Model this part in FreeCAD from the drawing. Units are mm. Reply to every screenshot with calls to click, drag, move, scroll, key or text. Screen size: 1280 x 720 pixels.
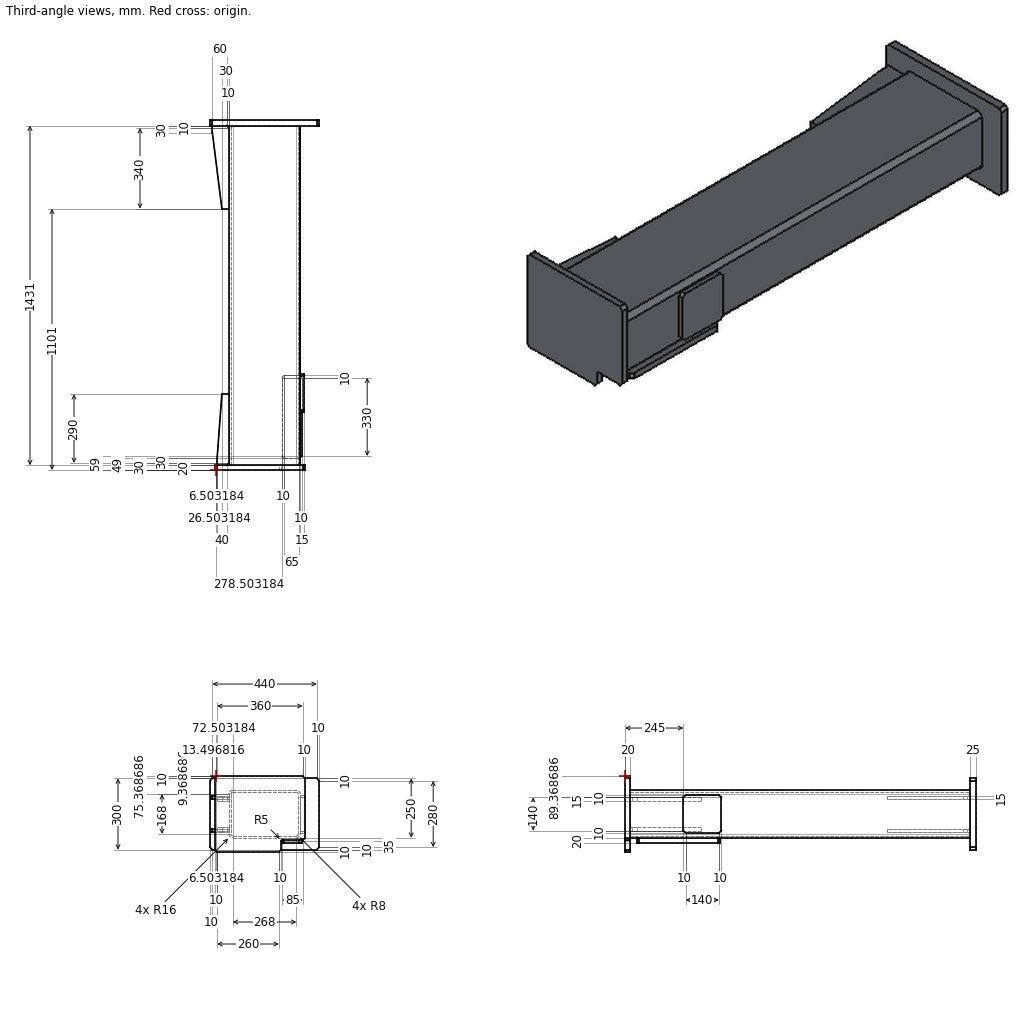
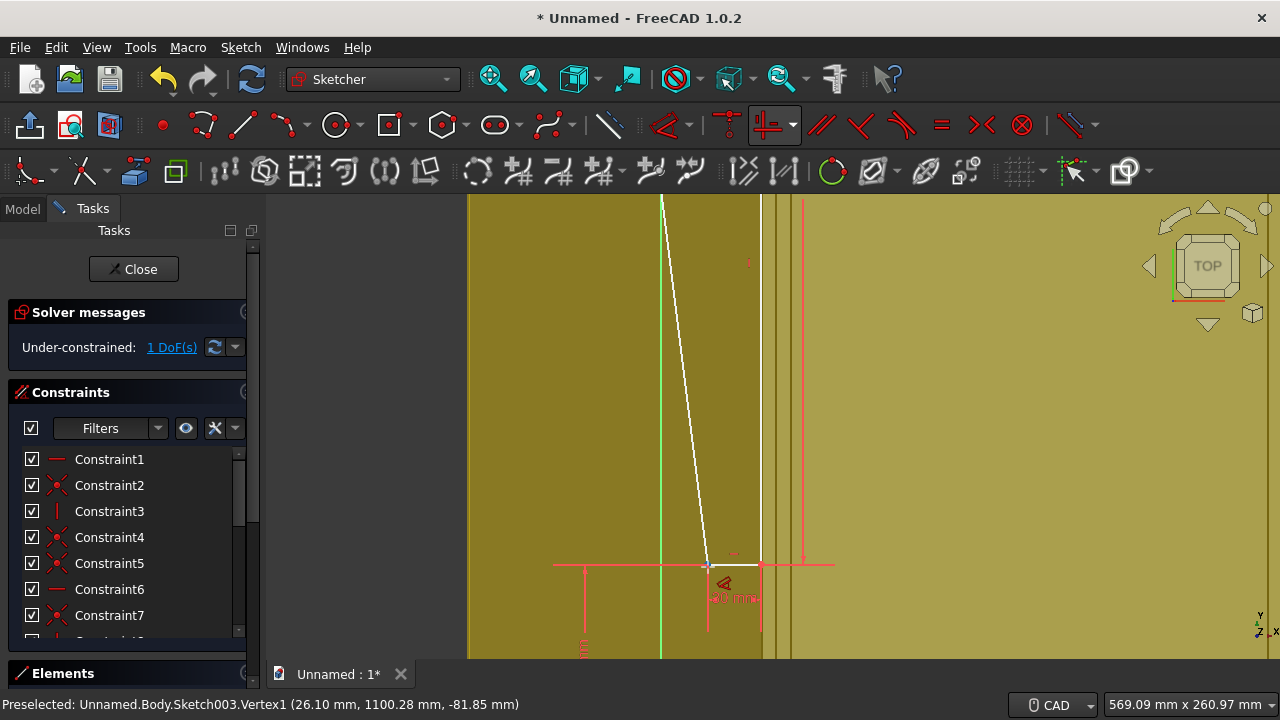
click(708, 565)
click(685, 531)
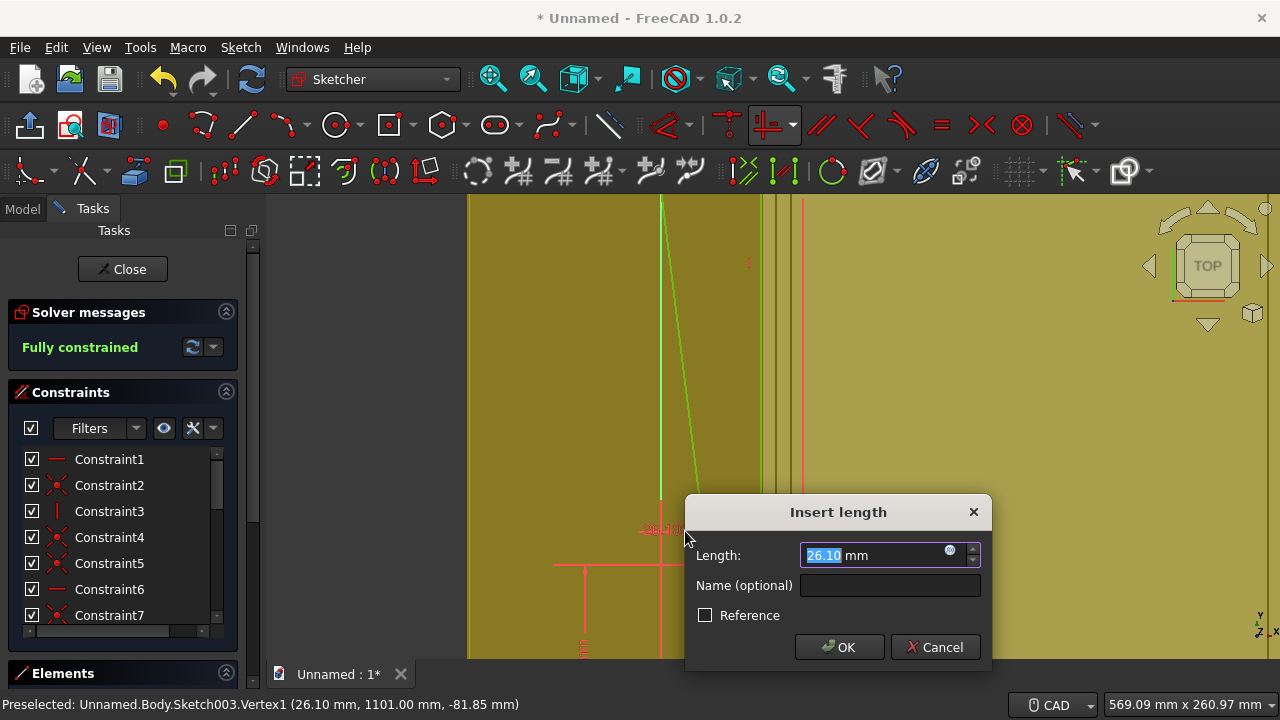
text(26.503184)
key(Return)
key(Escape)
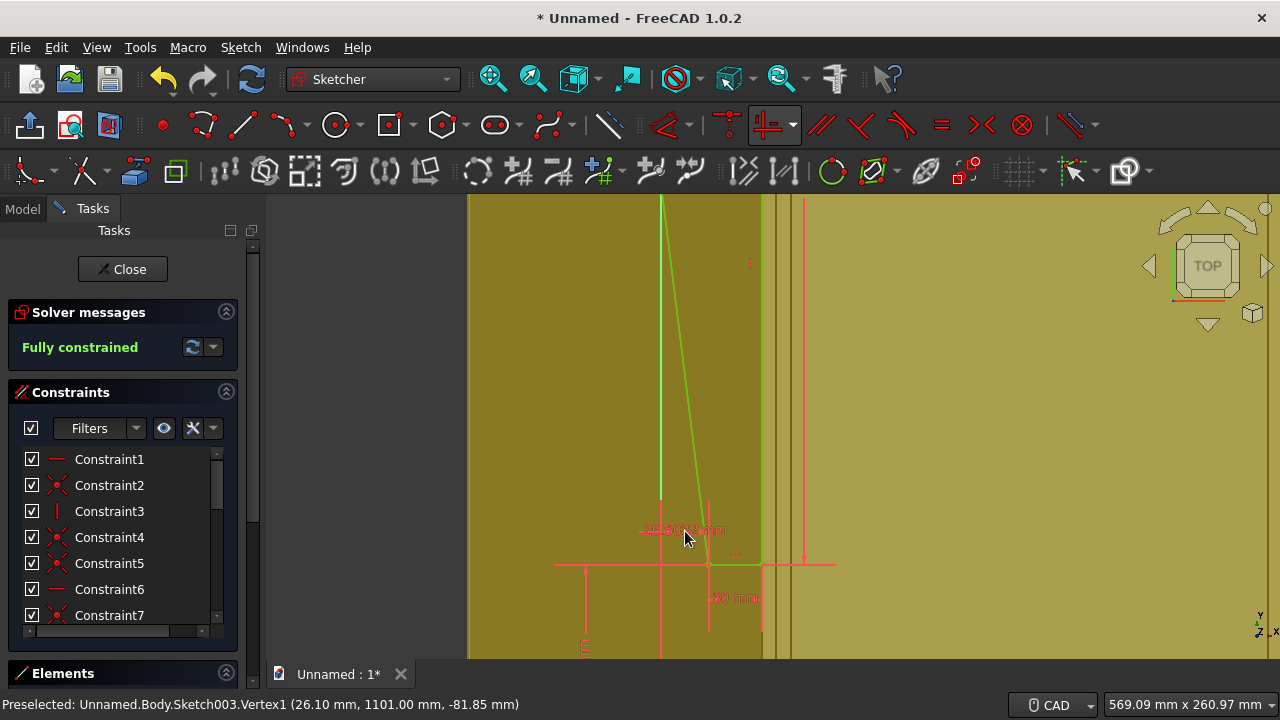
click(123, 269)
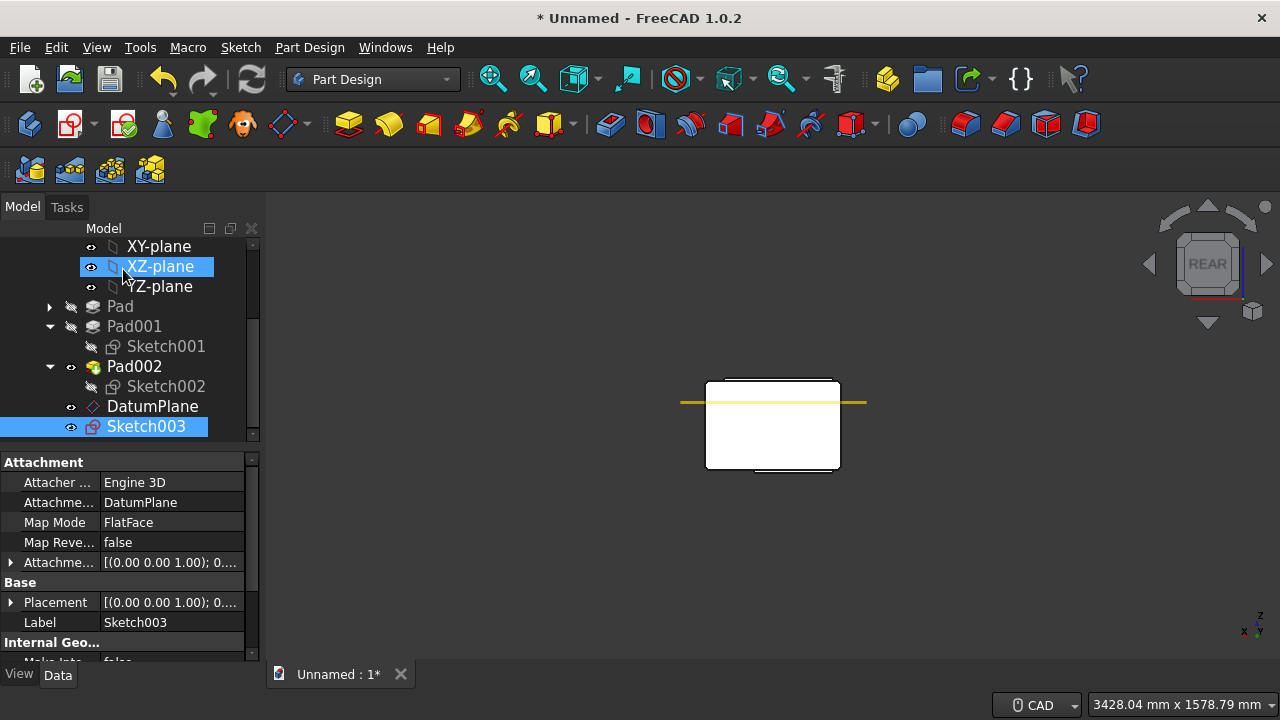
click(350, 124)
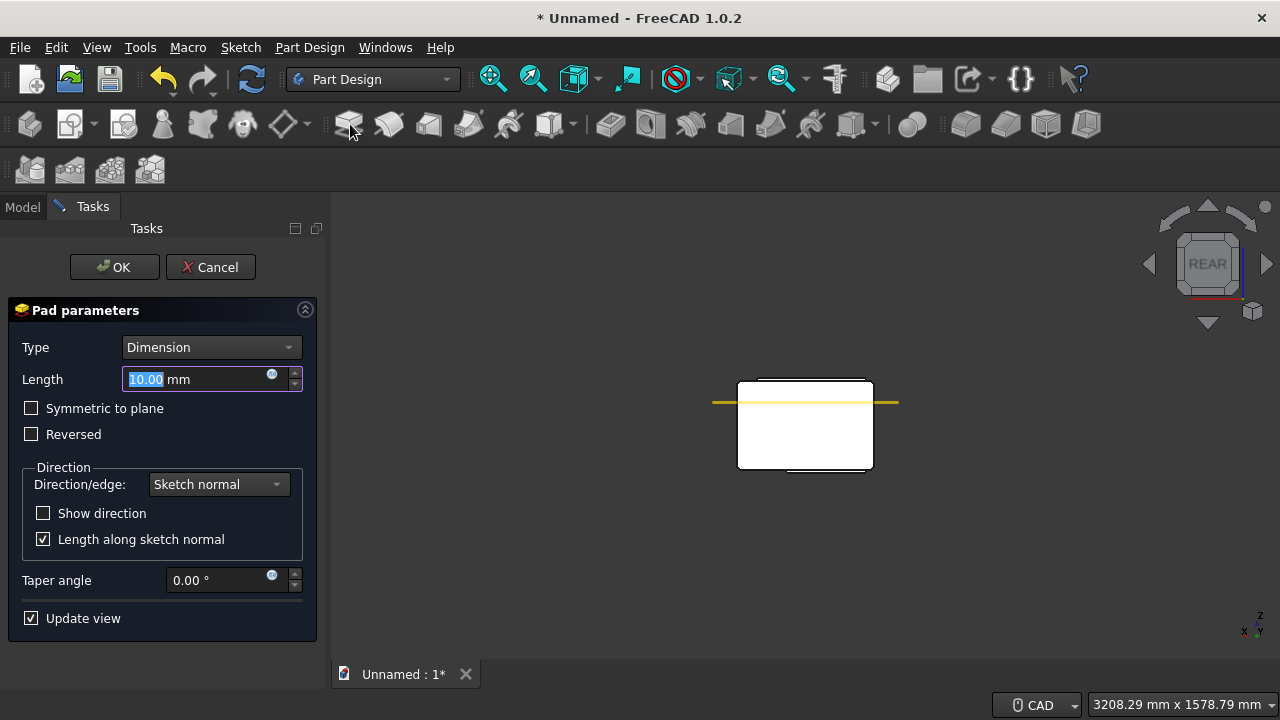
text(15)
key(Tab)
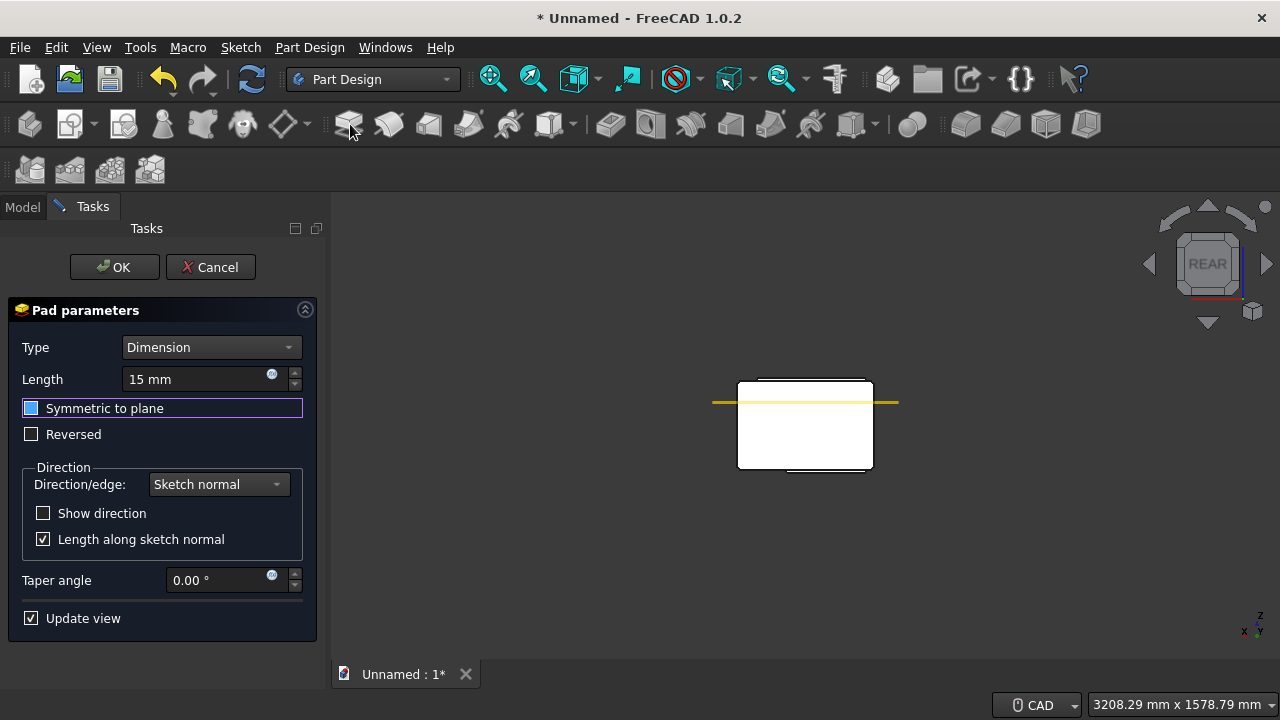
click(30, 434)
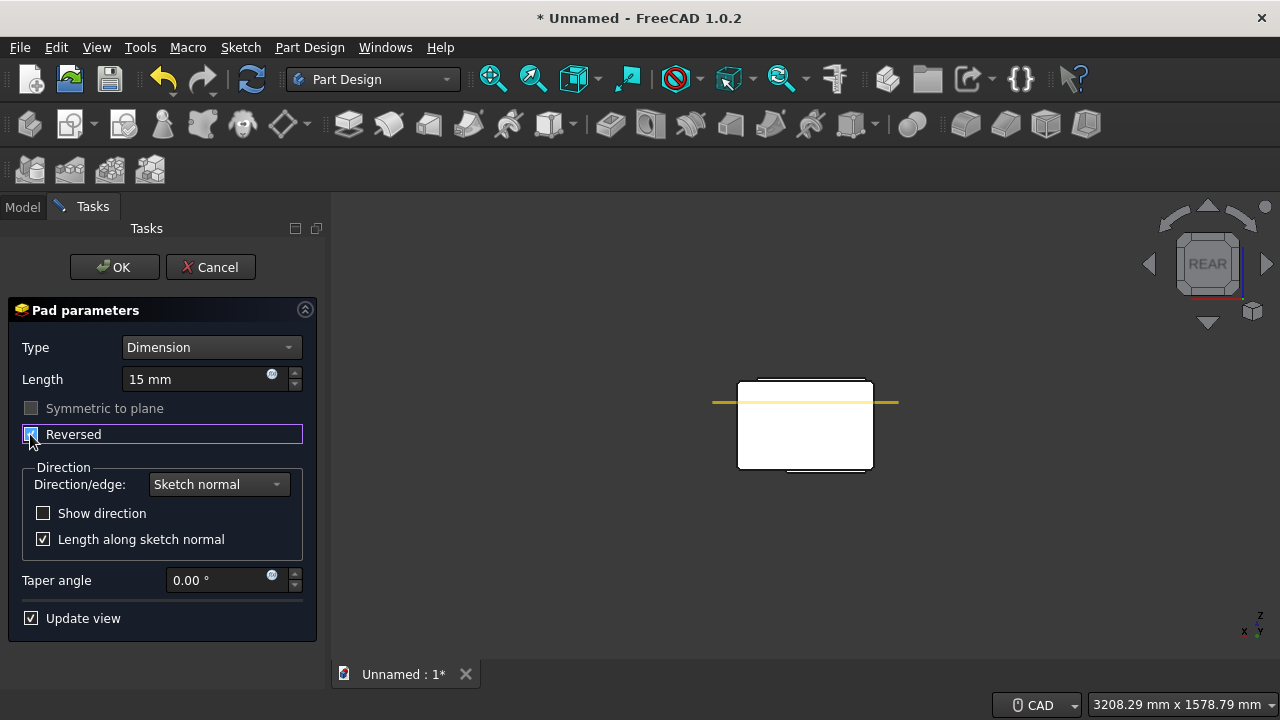
click(115, 267)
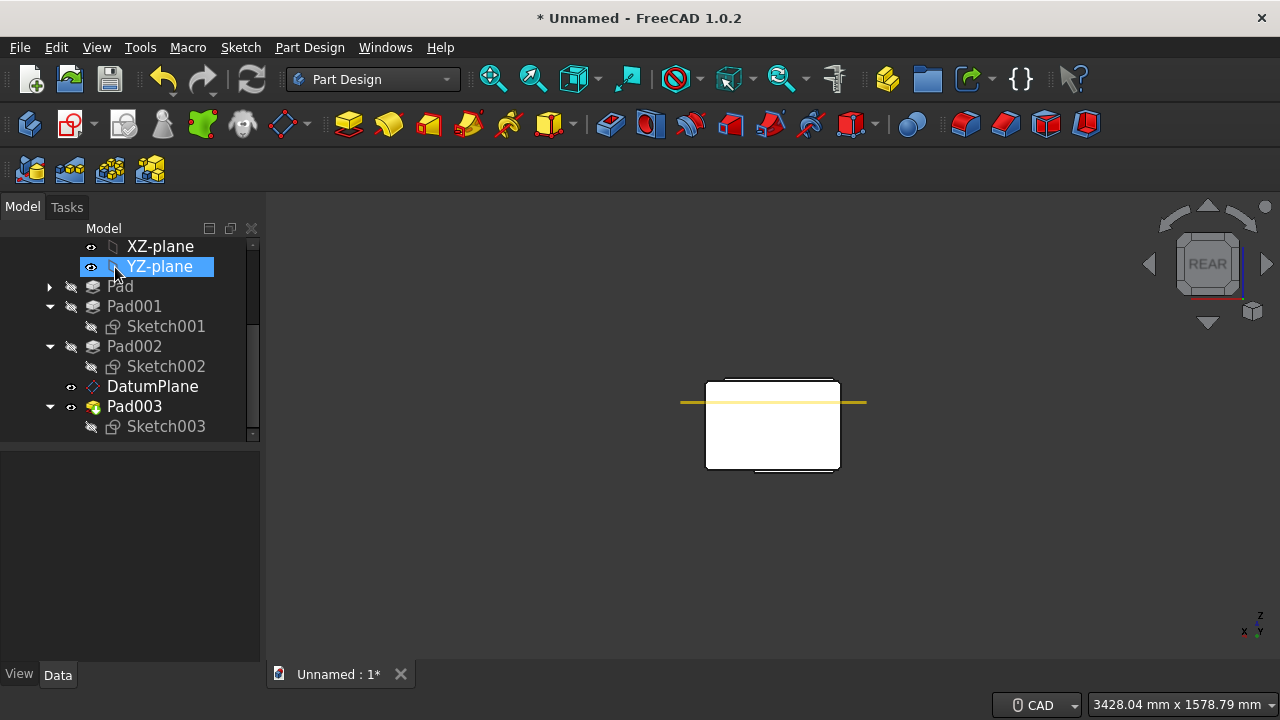
click(116, 387)
key(space)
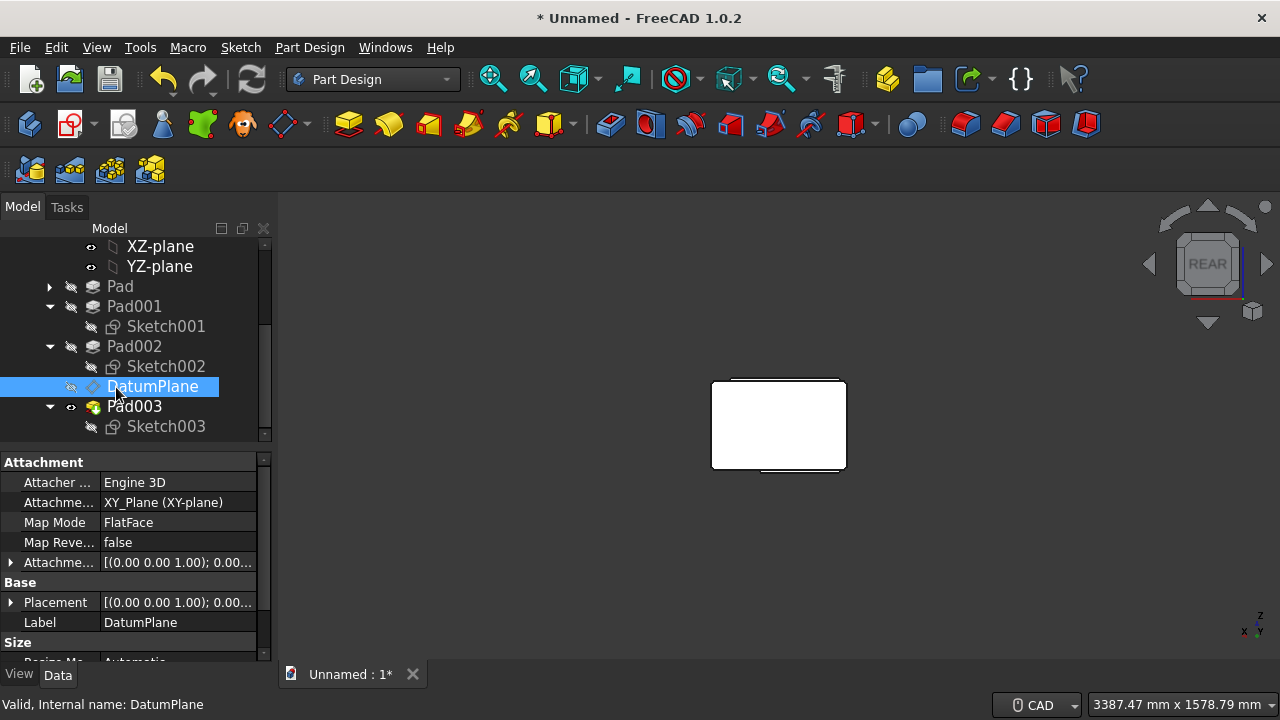
key(v)
key(f)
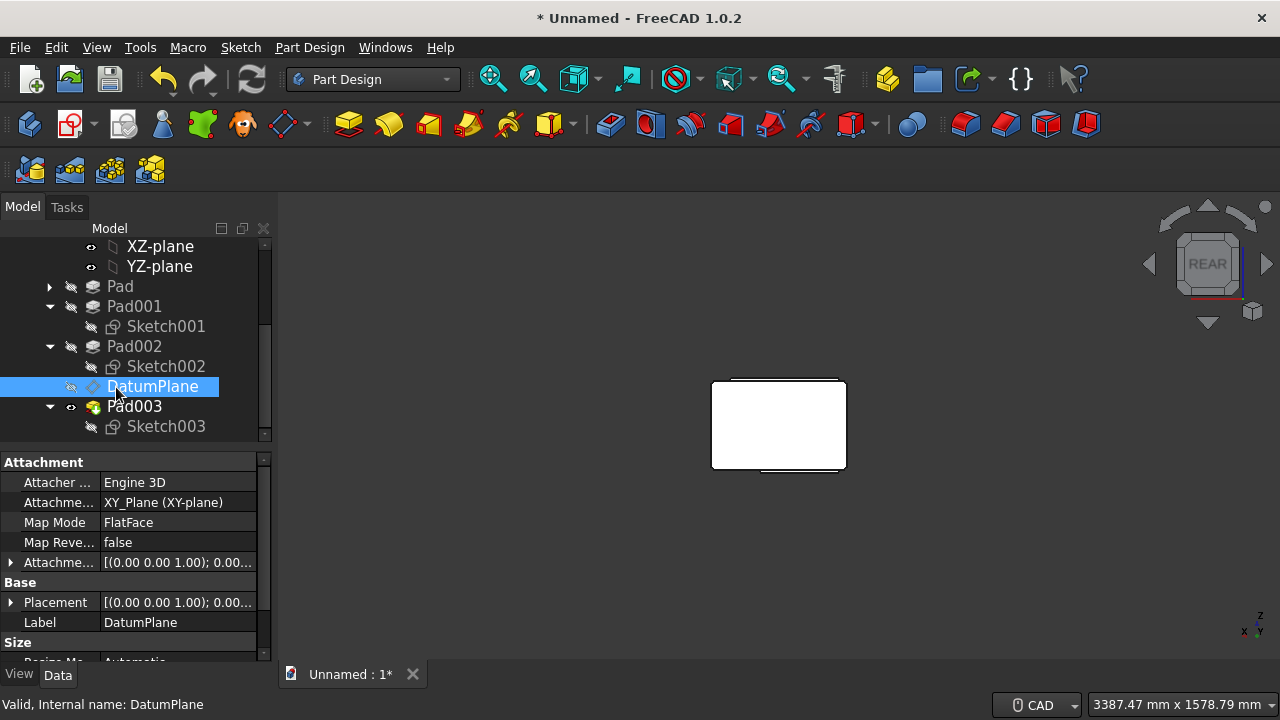
scroll(160, 342, down, 3)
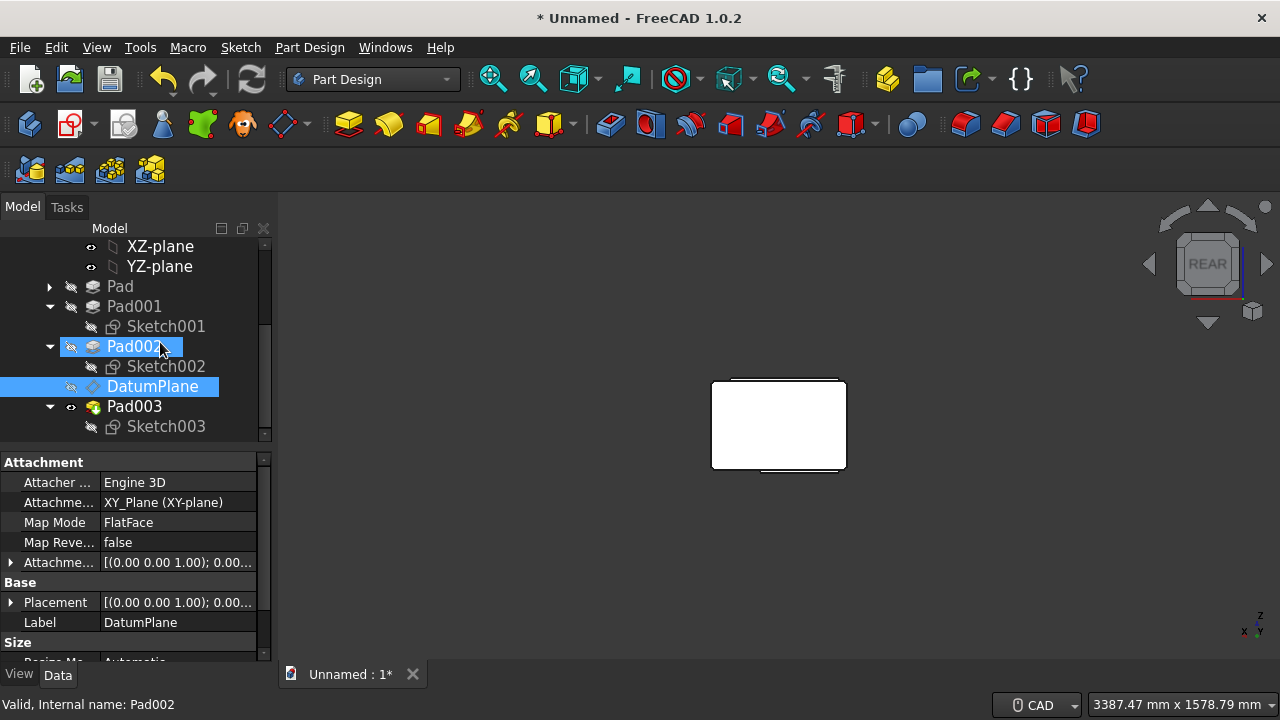
scroll(160, 342, up, 15)